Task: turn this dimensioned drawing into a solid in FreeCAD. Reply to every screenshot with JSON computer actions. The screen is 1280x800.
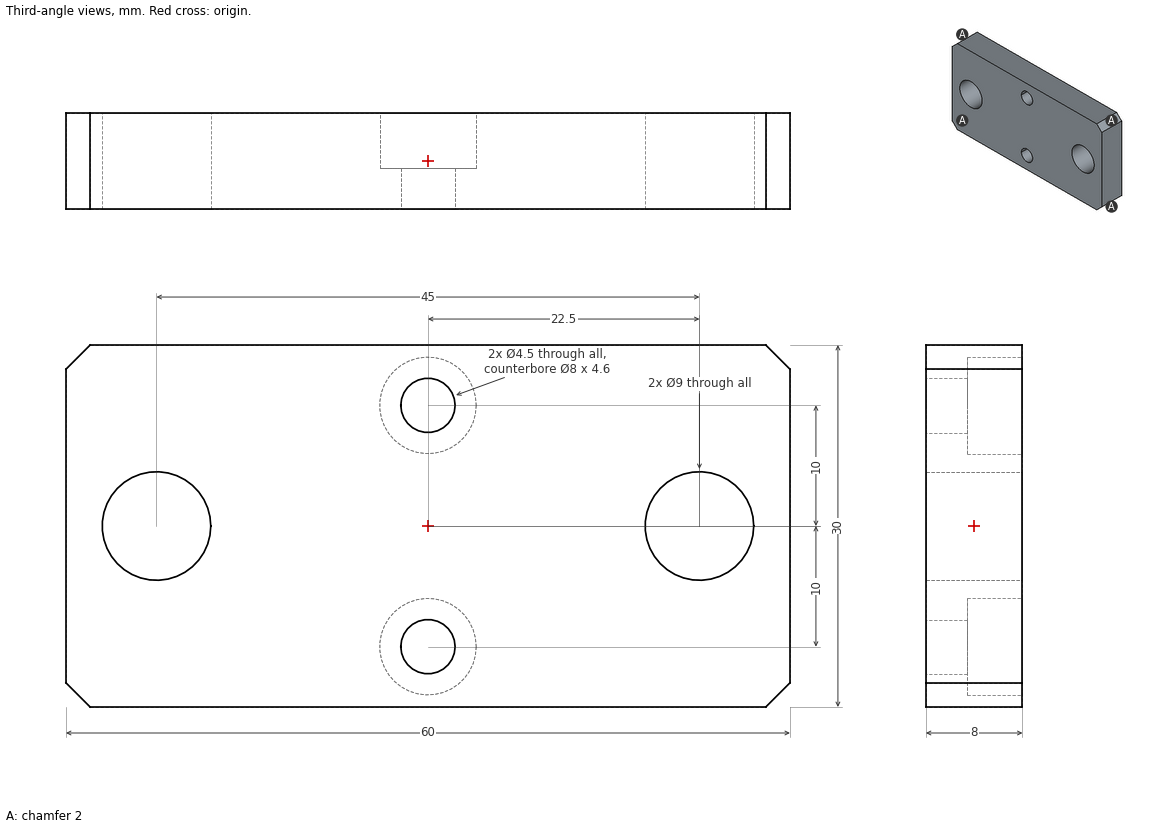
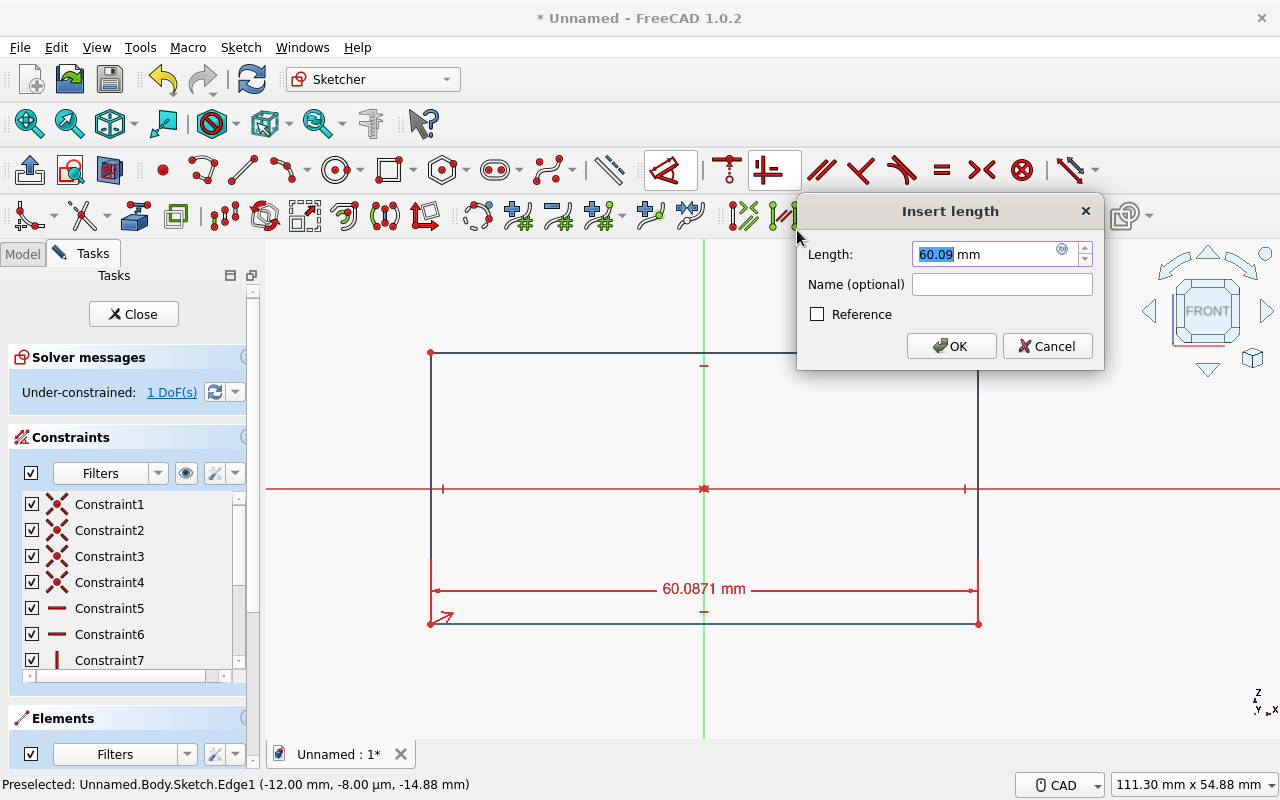
{"action": "type", "text": "60"}
{"action": "key", "text": "Return"}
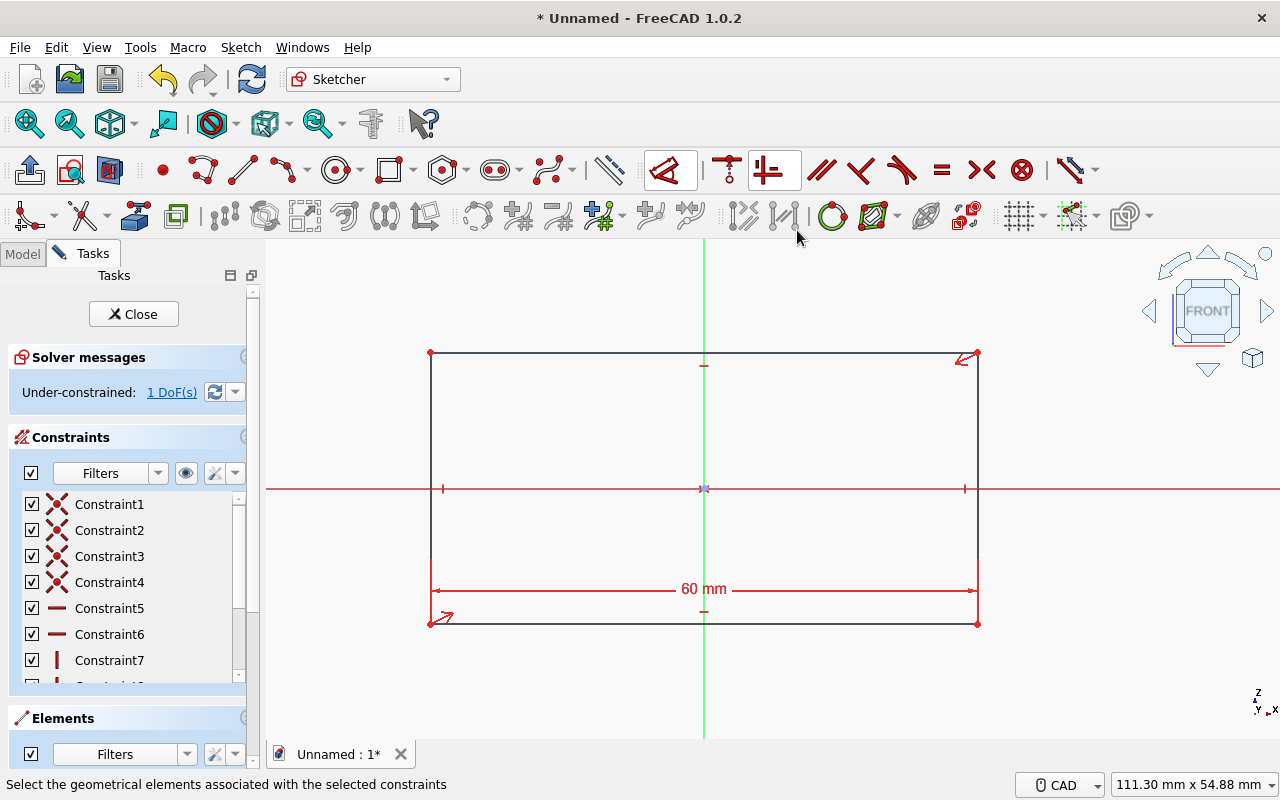
{"action": "left_click", "coordinate": [978, 543]}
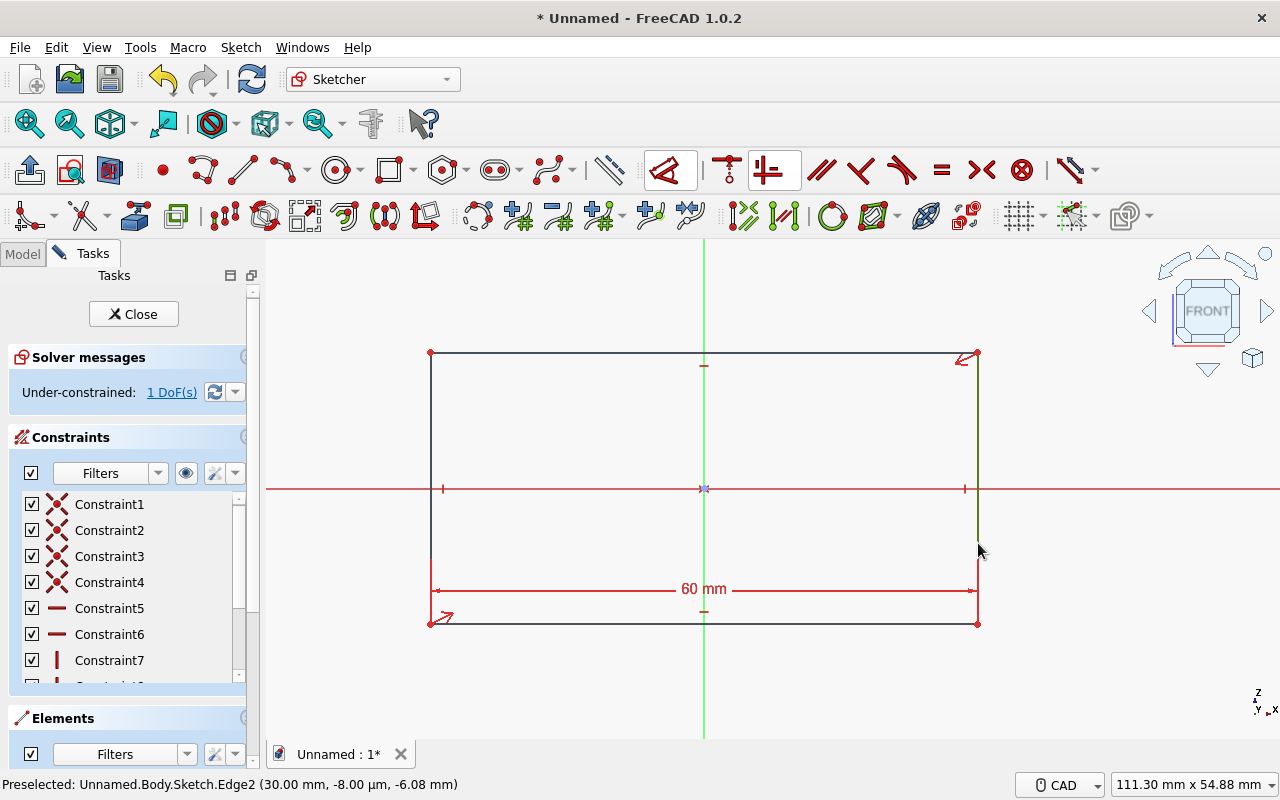
{"action": "left_click", "coordinate": [692, 170]}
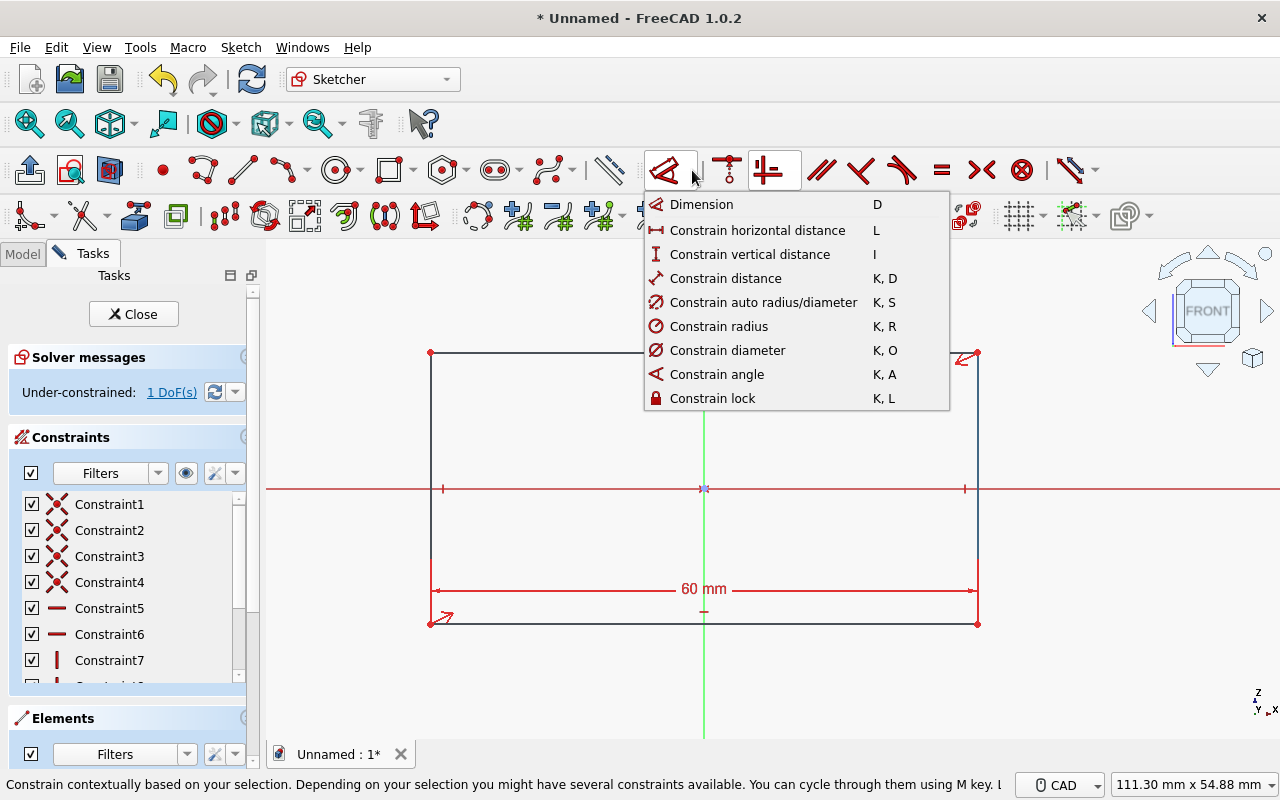
{"action": "left_click", "coordinate": [797, 254]}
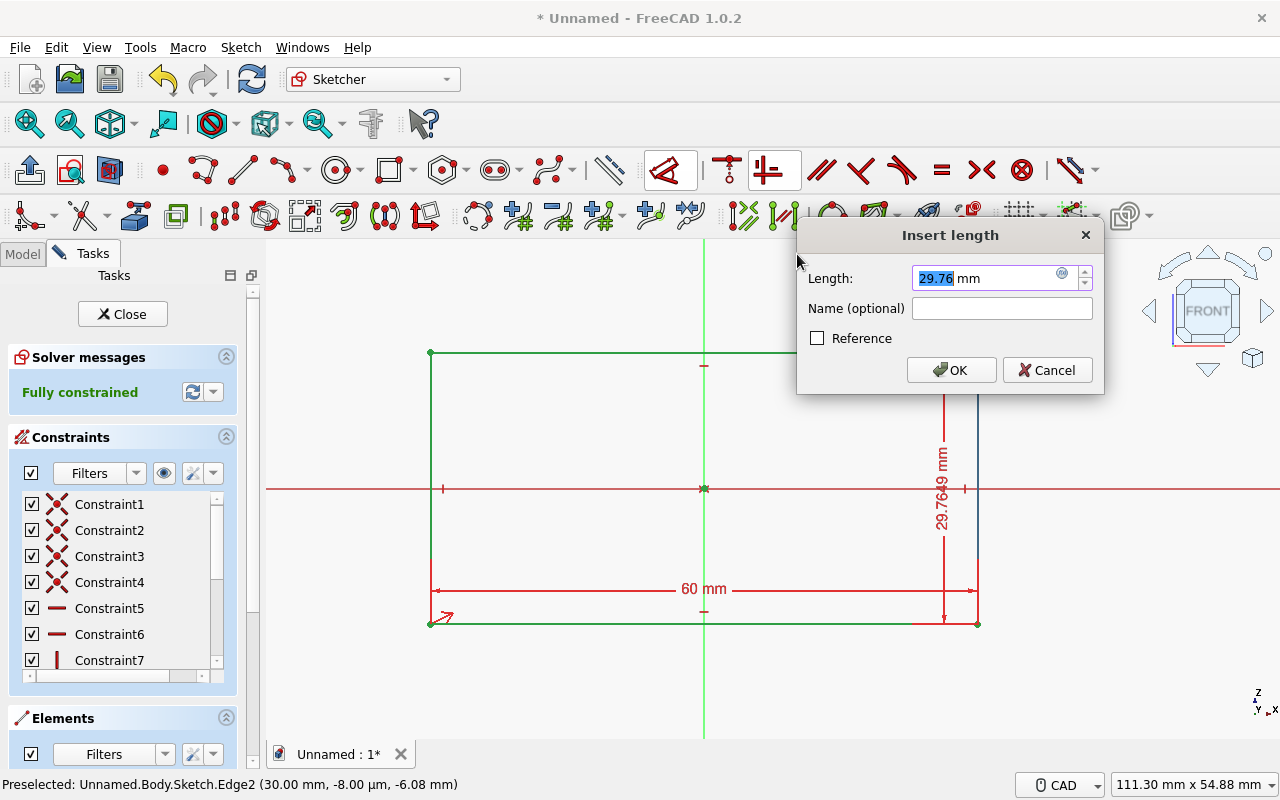
{"action": "type", "text": "30"}
{"action": "key", "text": "Return"}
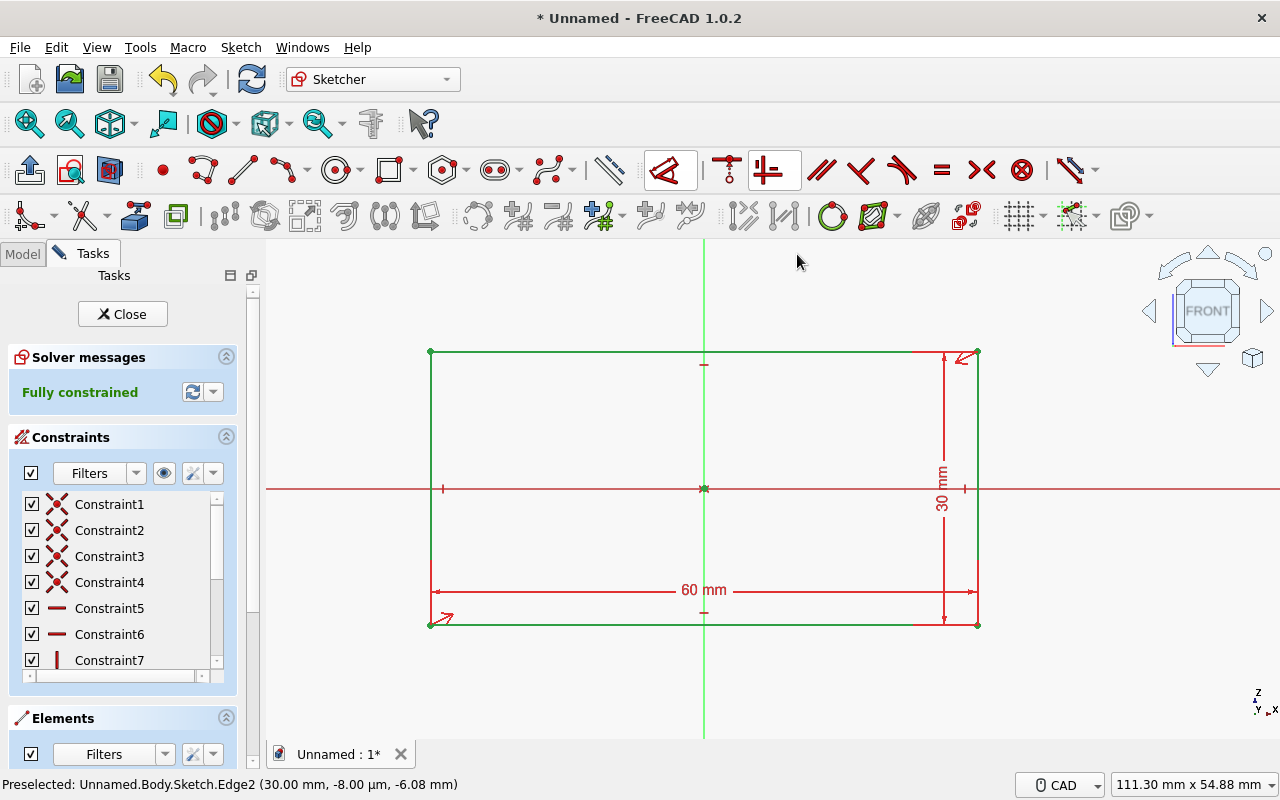
{"action": "left_click", "coordinate": [123, 314]}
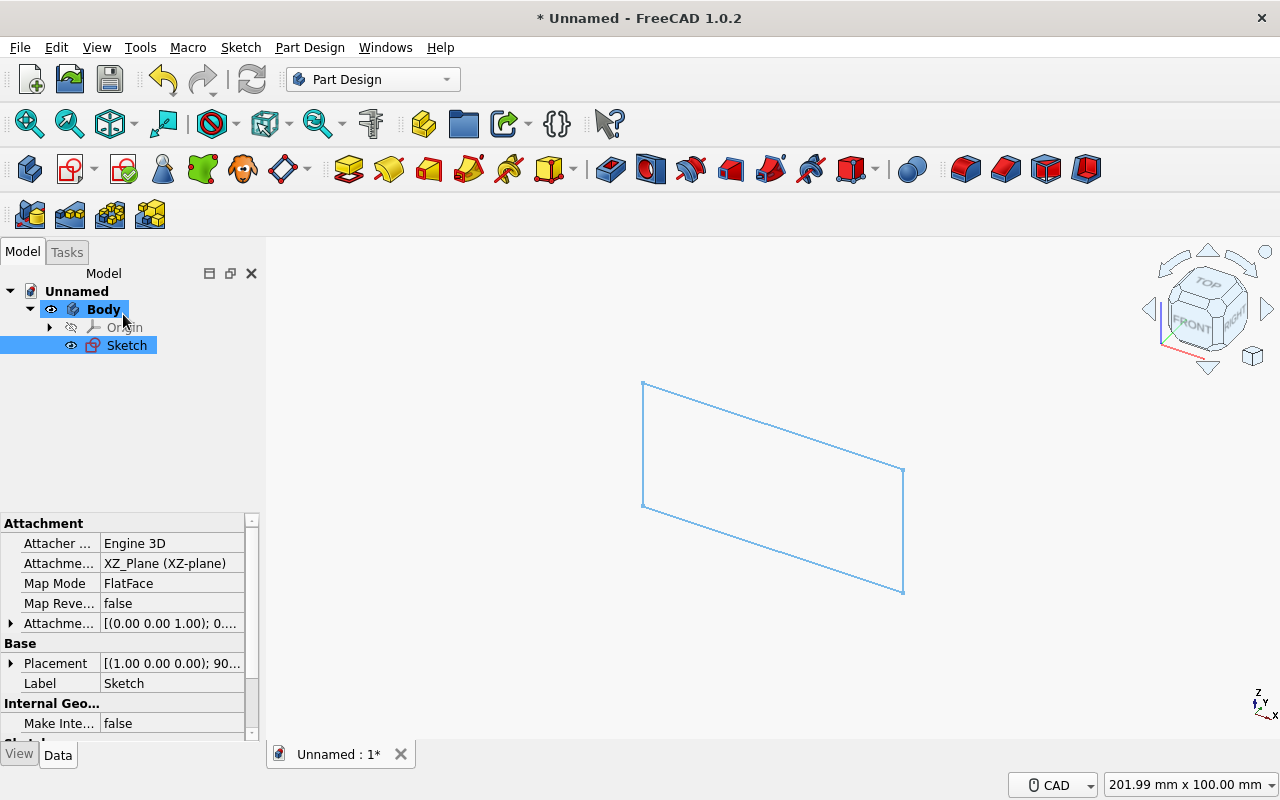
{"action": "left_click", "coordinate": [350, 170]}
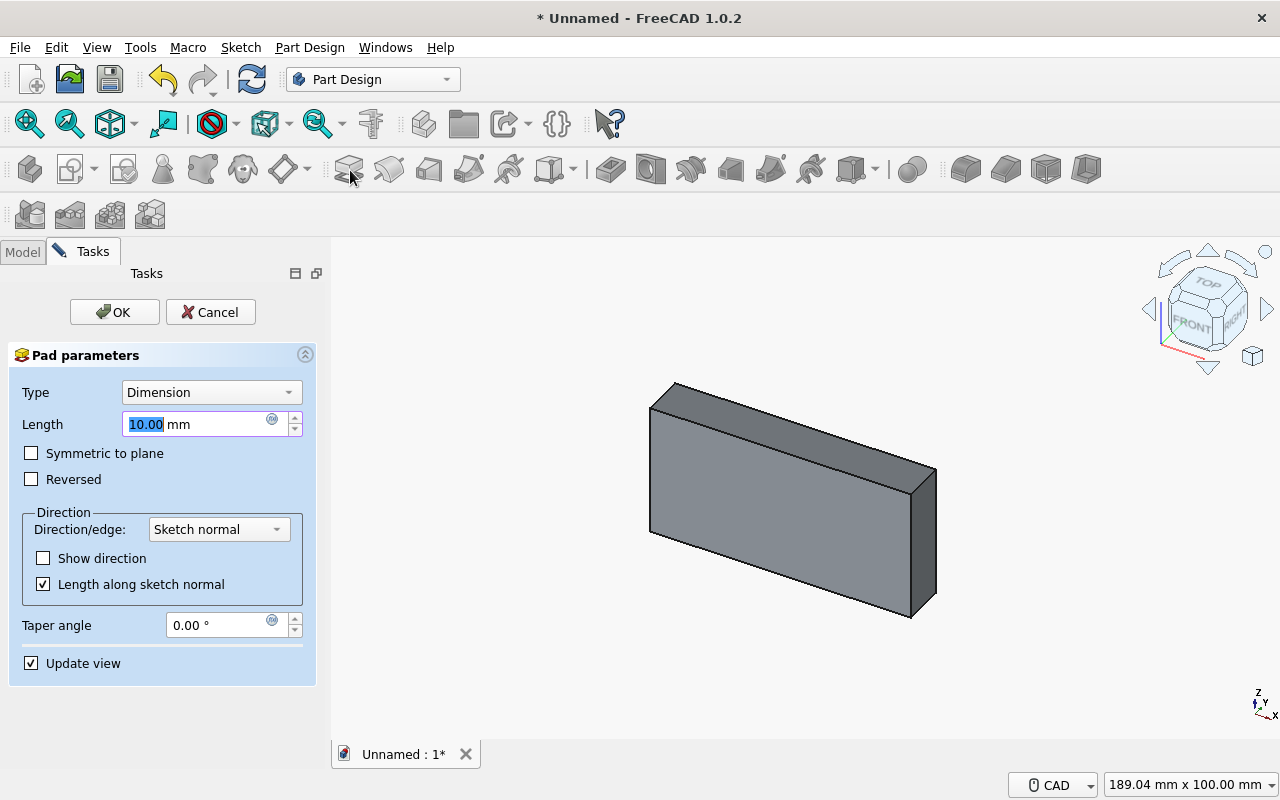
{"action": "type", "text": "8"}
{"action": "key", "text": "Tab"}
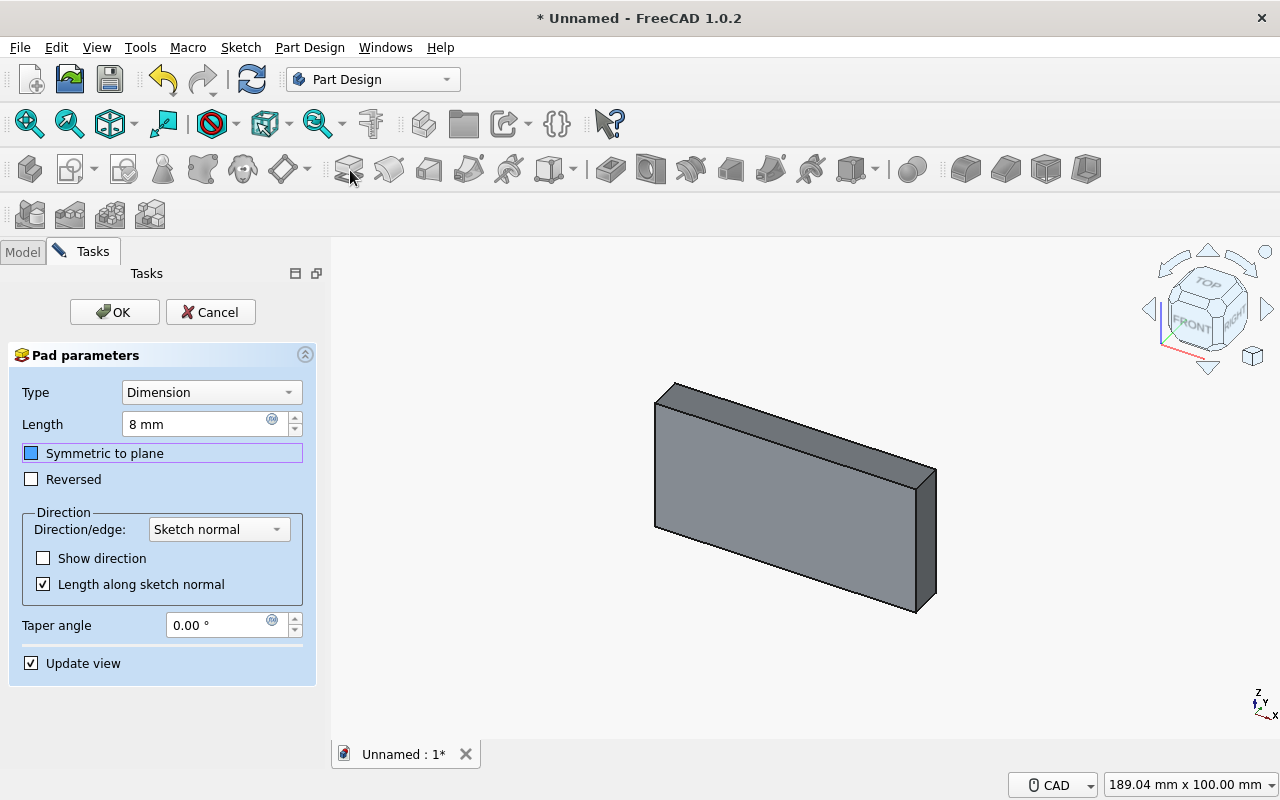
{"action": "left_click", "coordinate": [30, 453]}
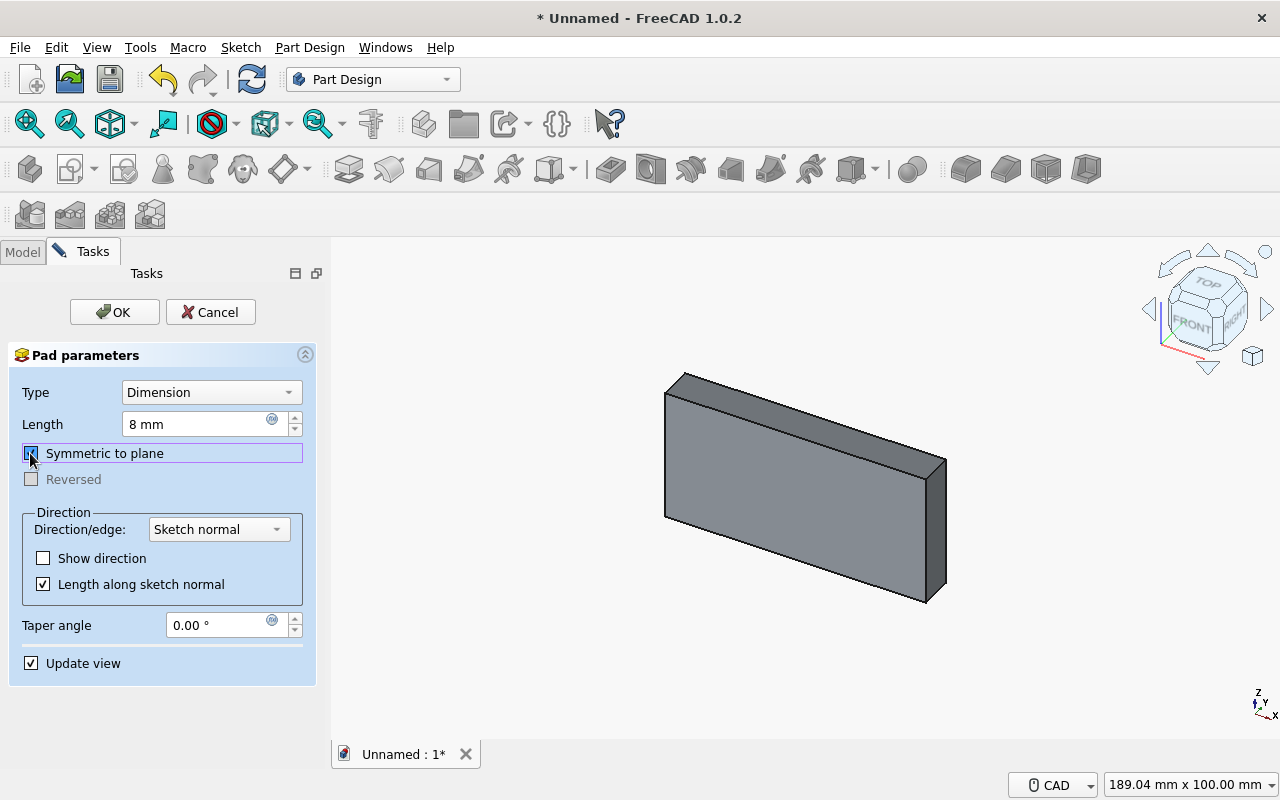
{"action": "left_click", "coordinate": [115, 312]}